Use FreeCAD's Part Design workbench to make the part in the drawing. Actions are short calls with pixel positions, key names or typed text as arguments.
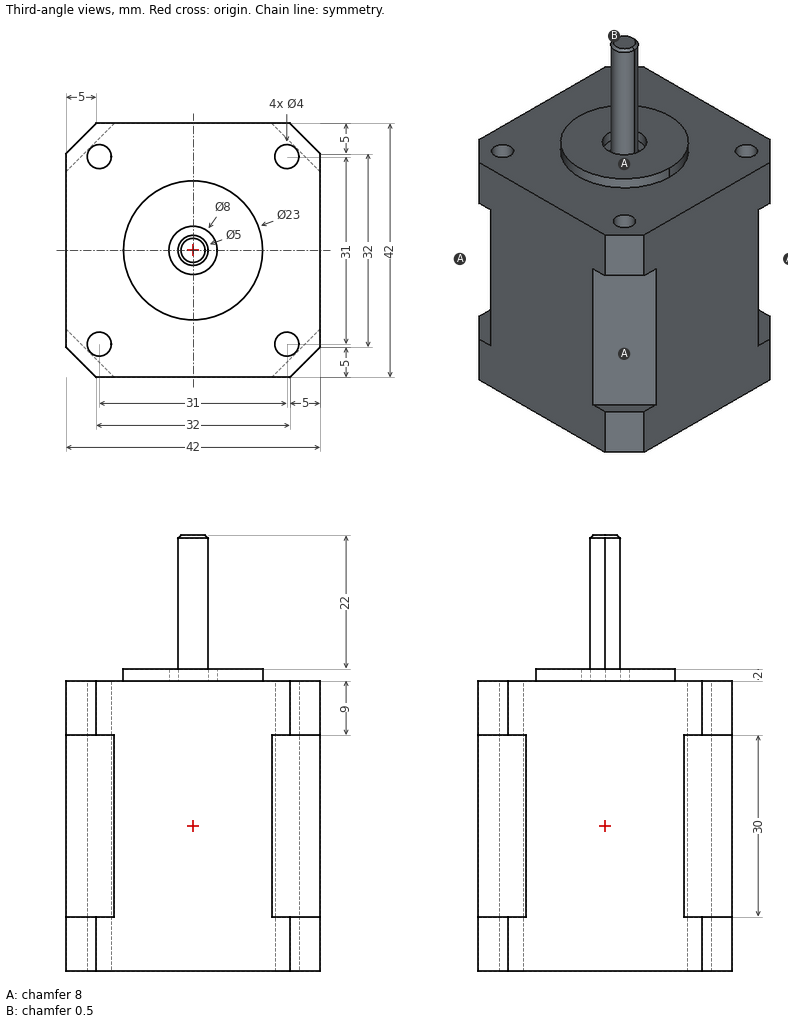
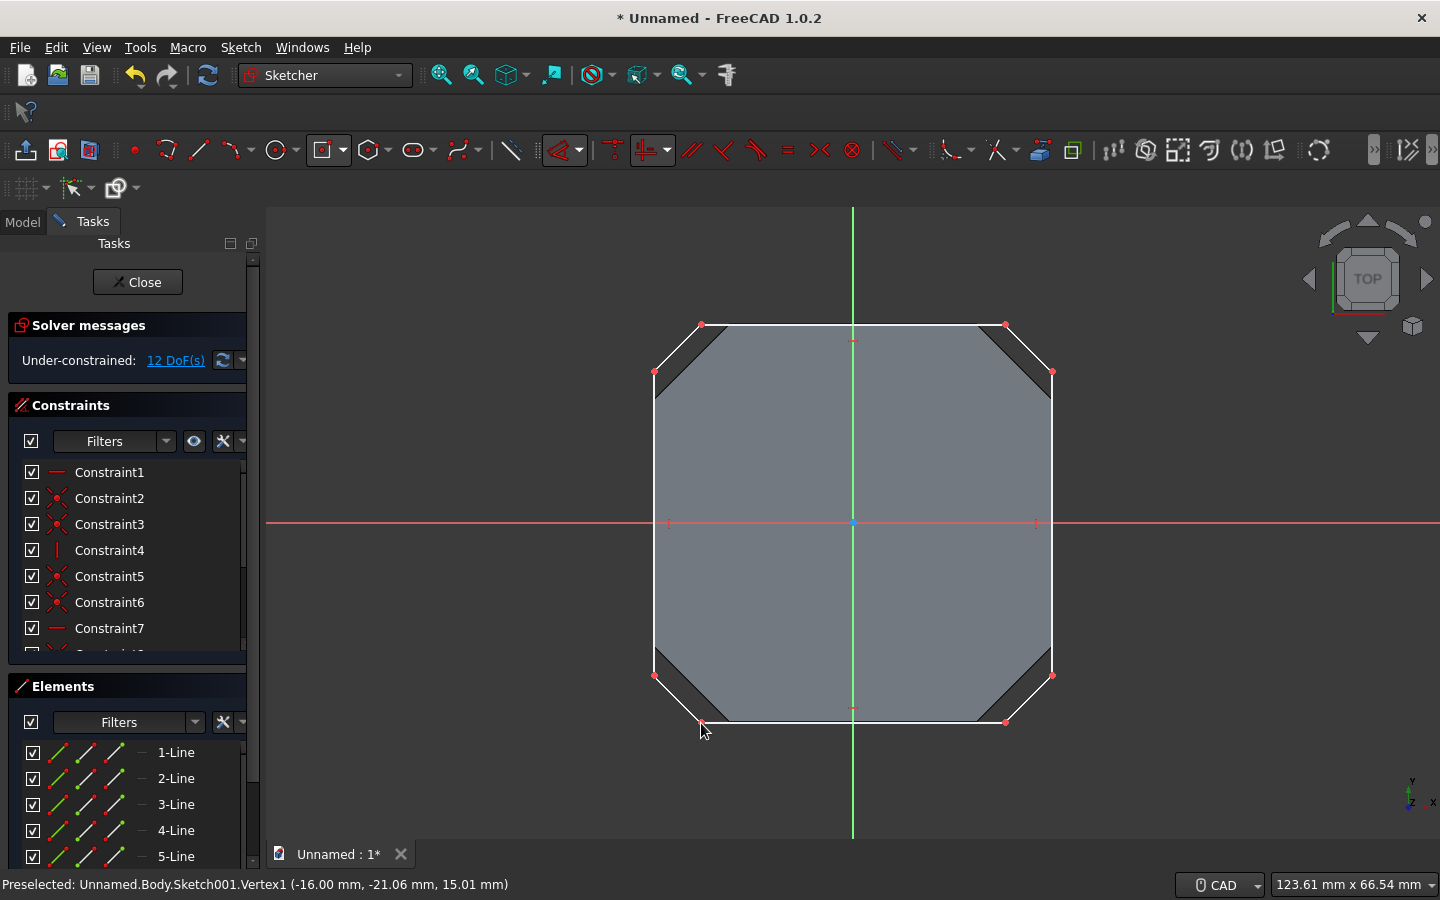
click(1005, 723)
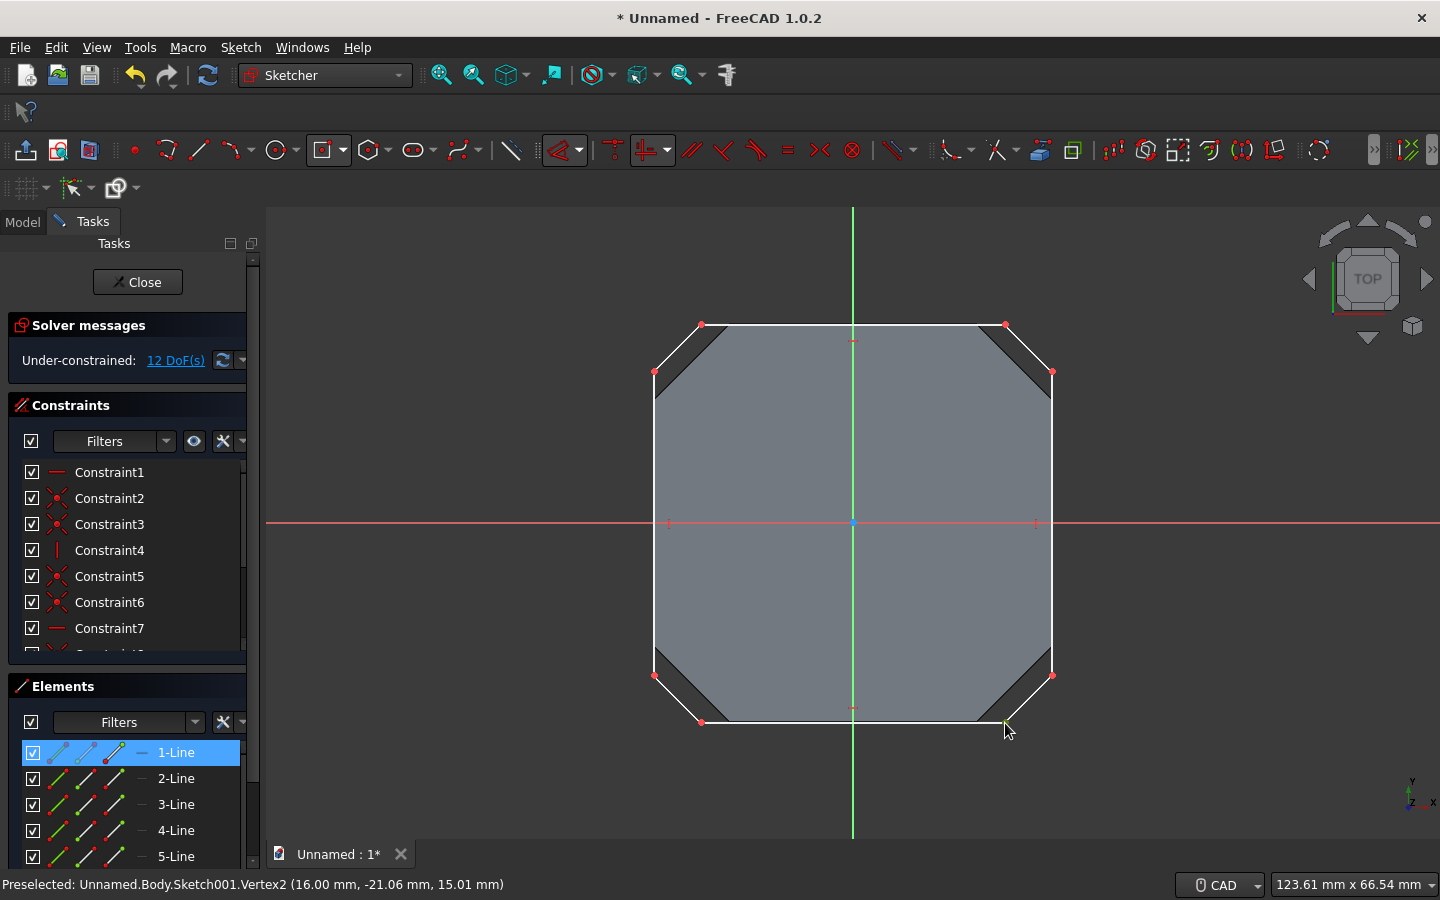
click(1005, 325)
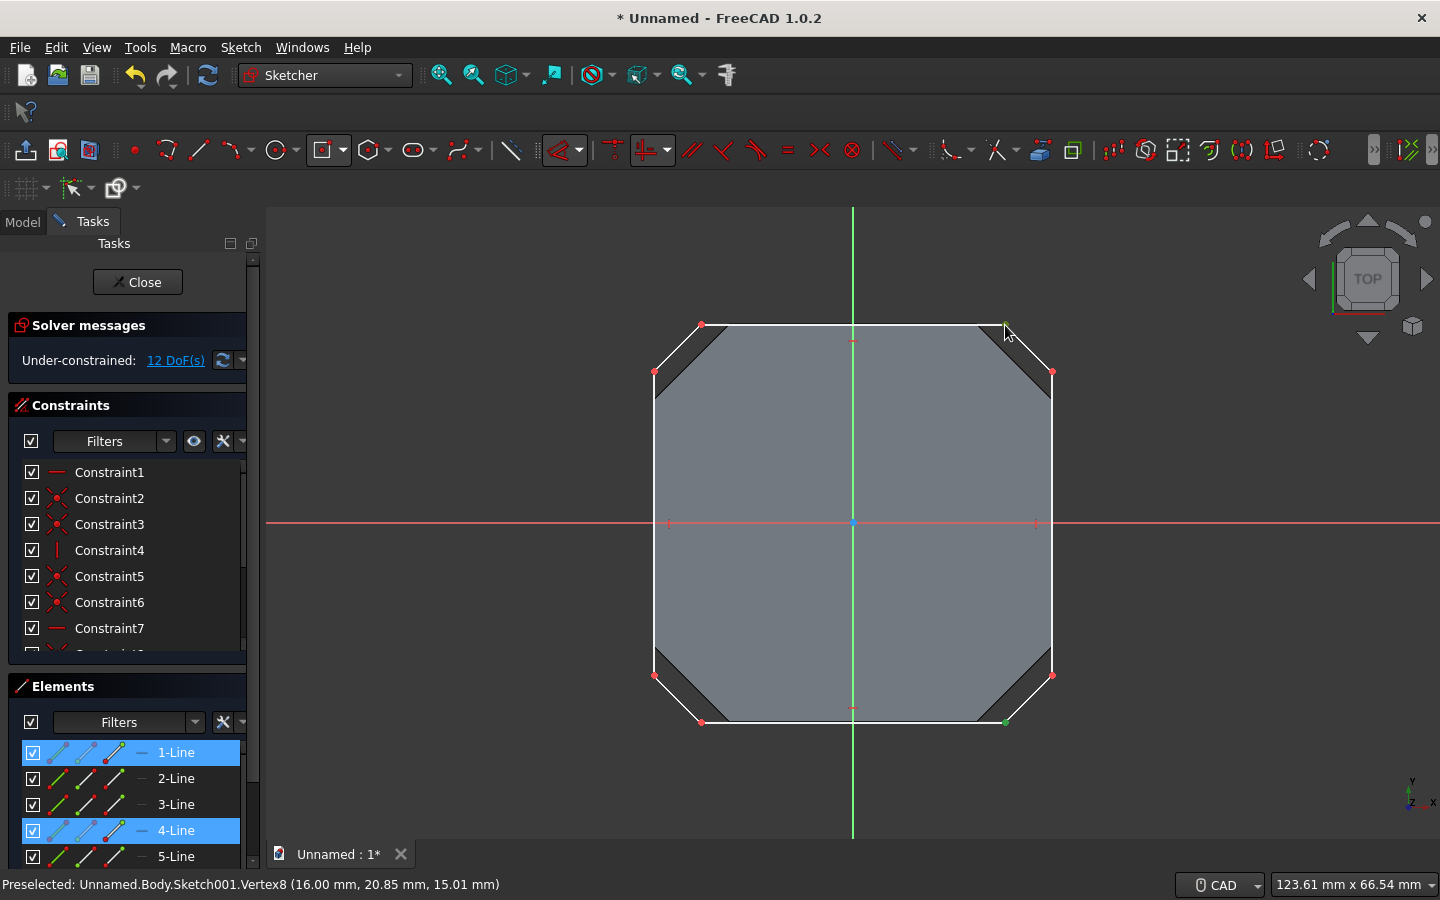
click(364, 523)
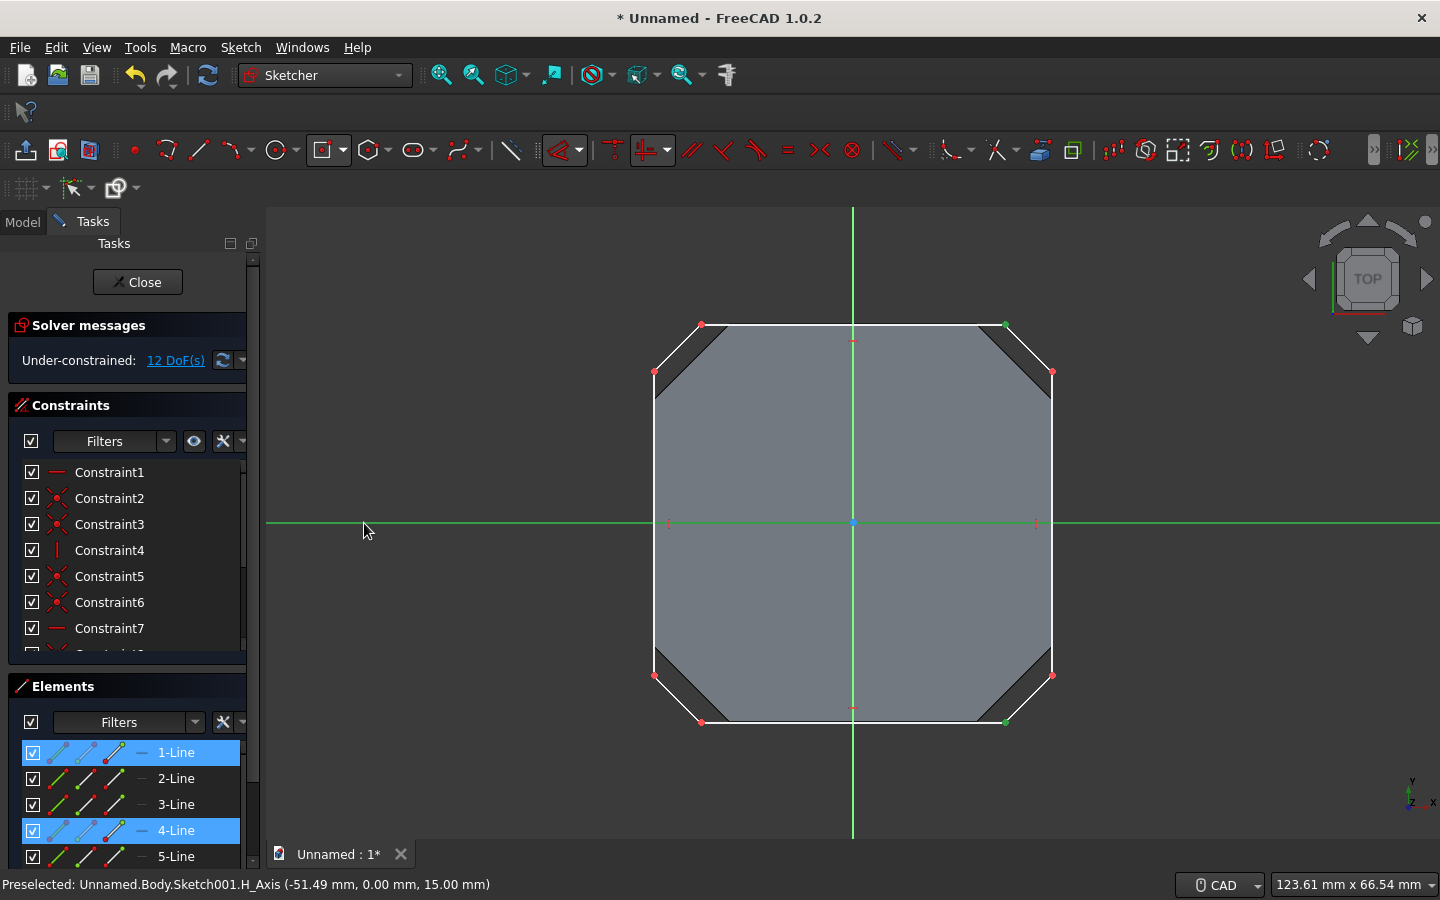
click(820, 150)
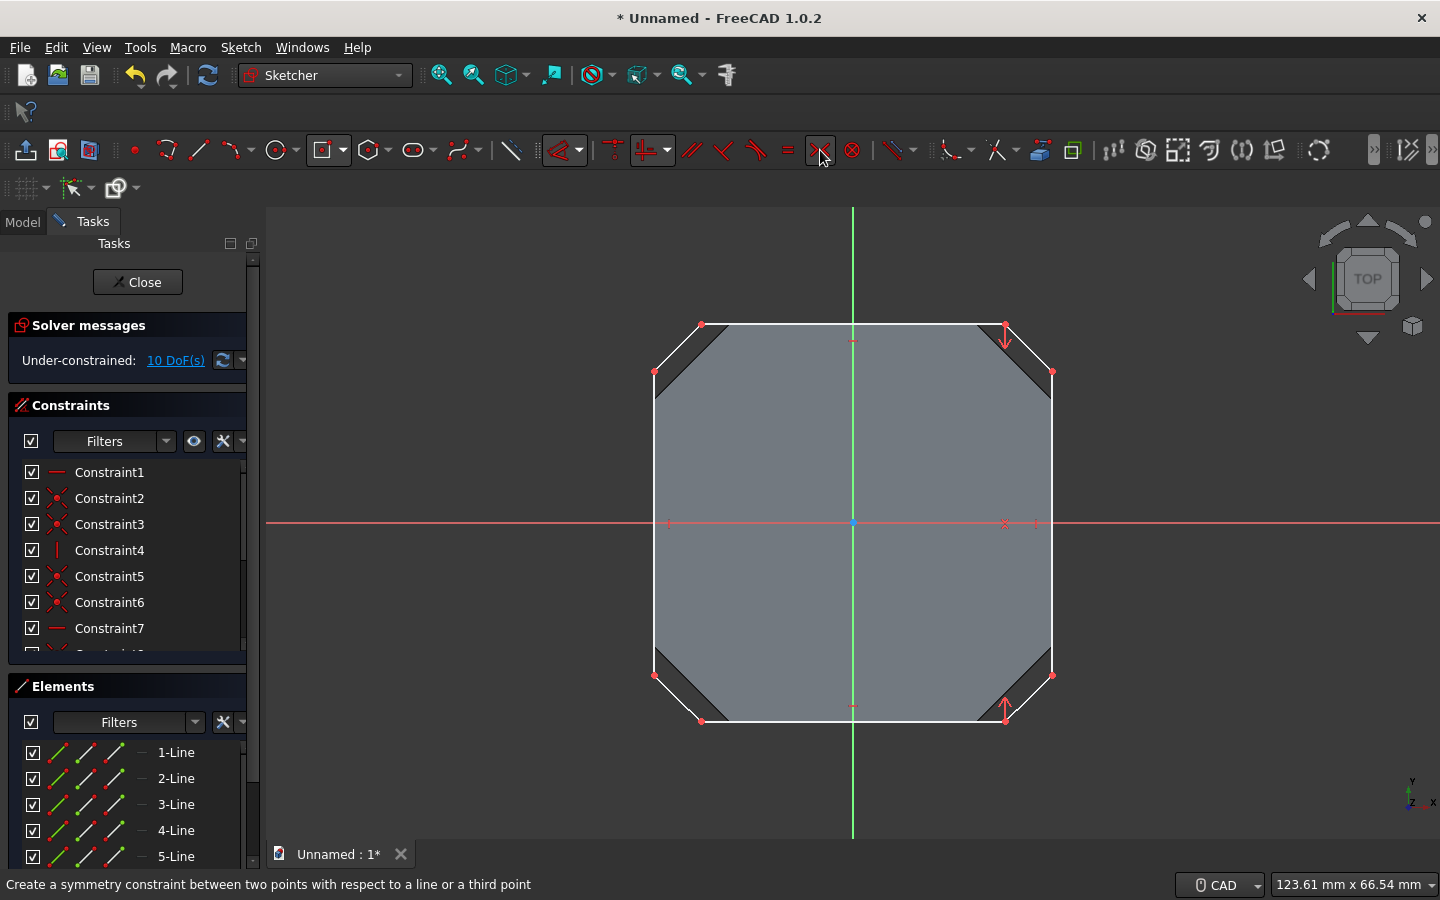
click(1052, 372)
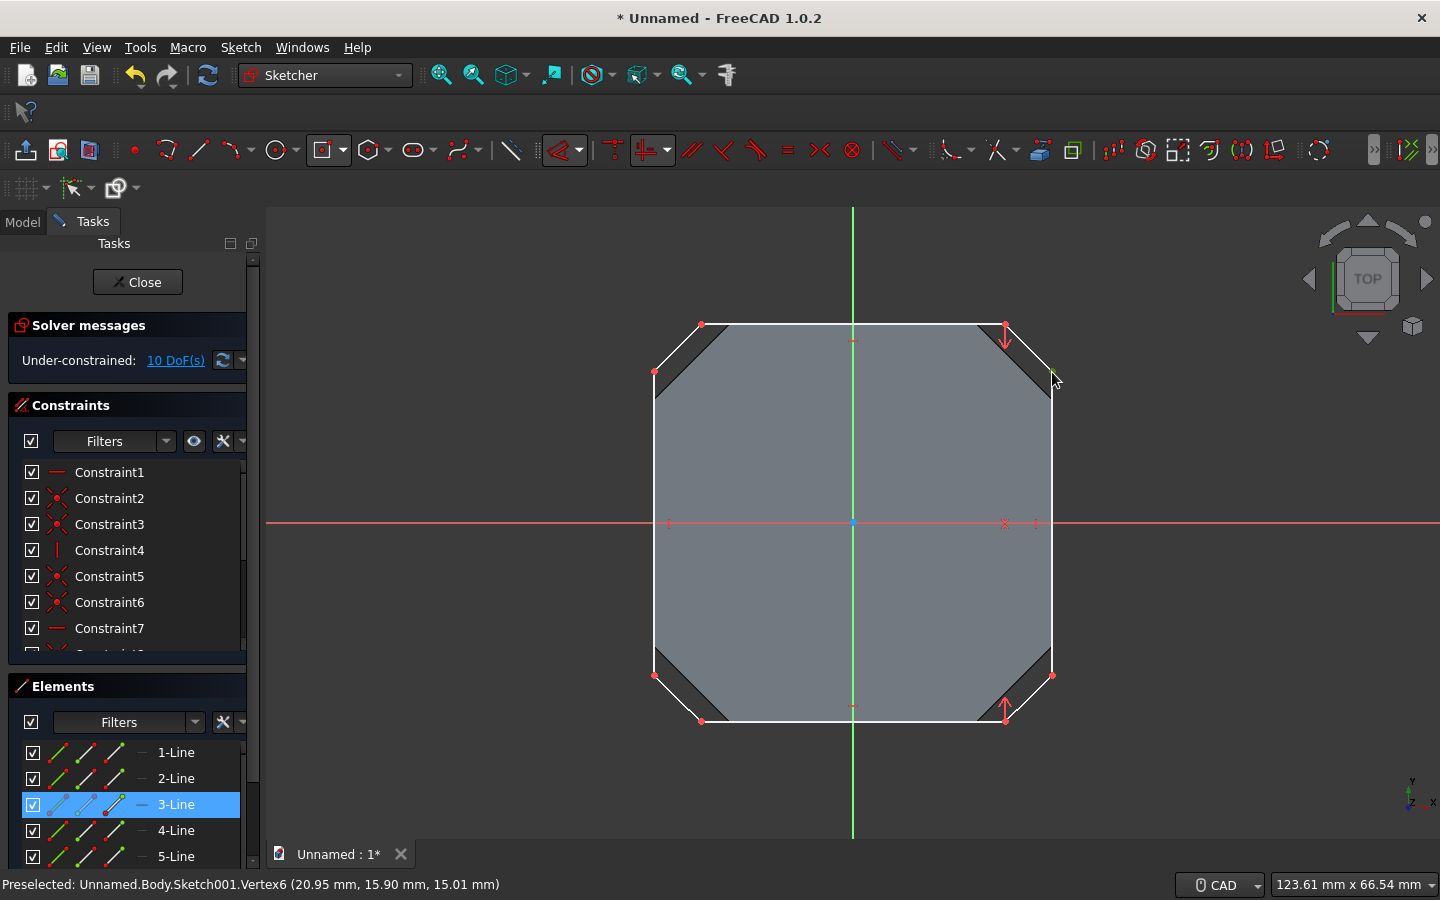
click(654, 372)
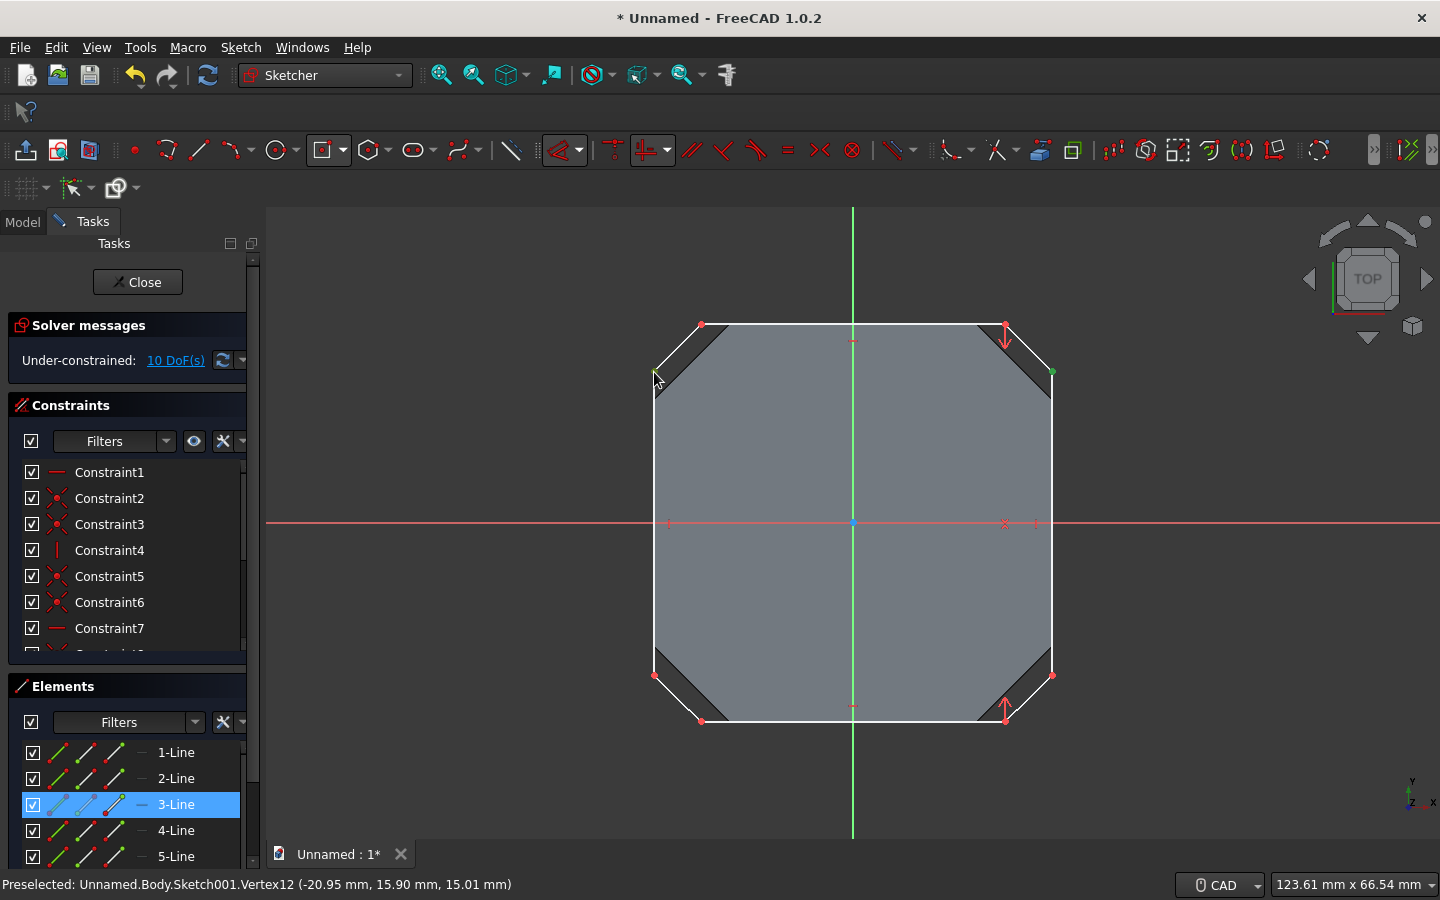
click(853, 770)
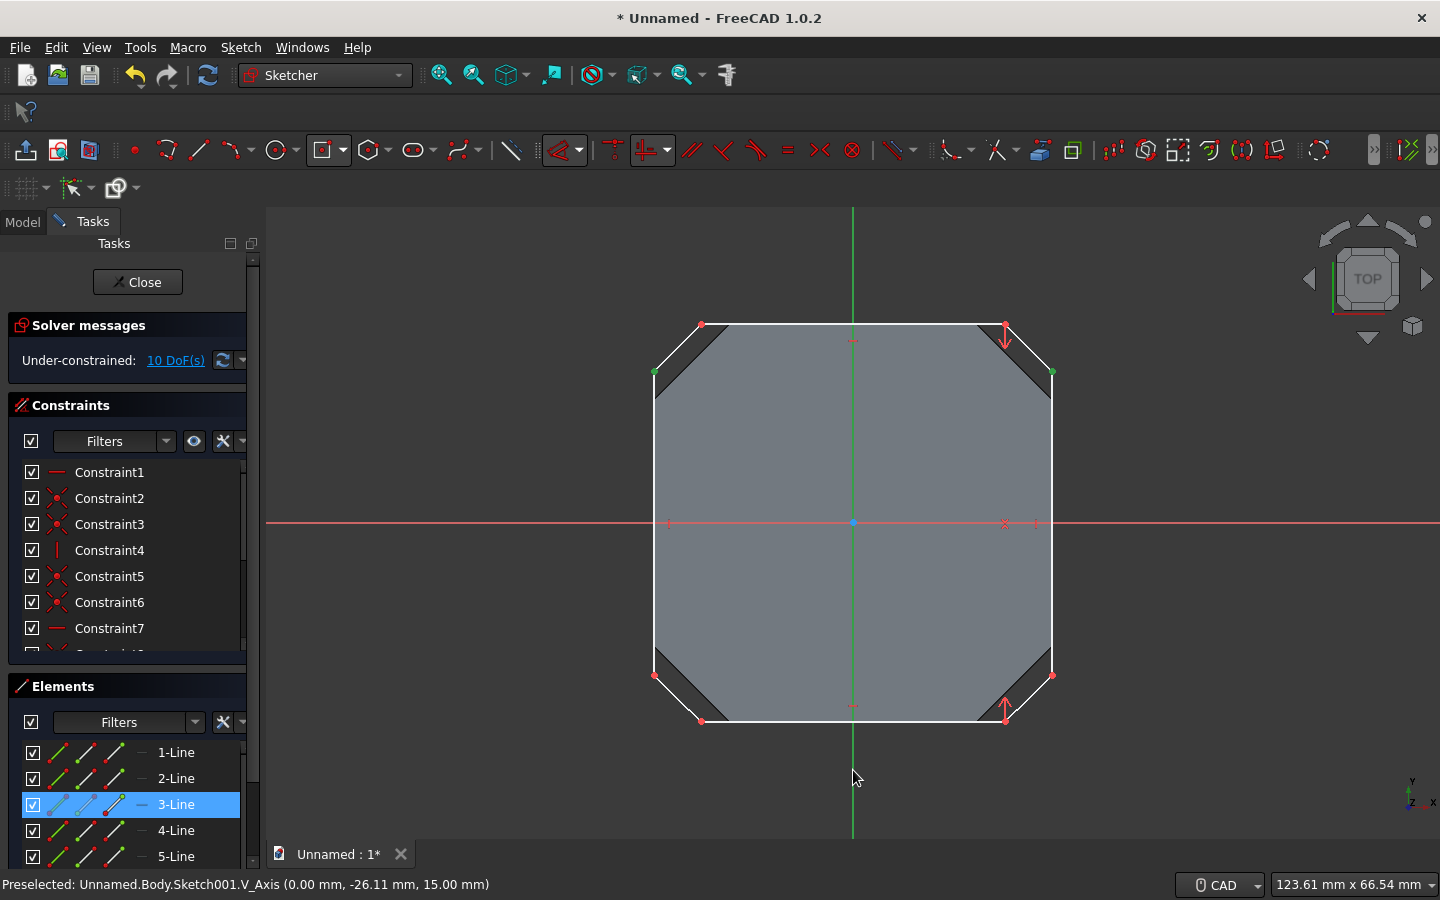
key(s)